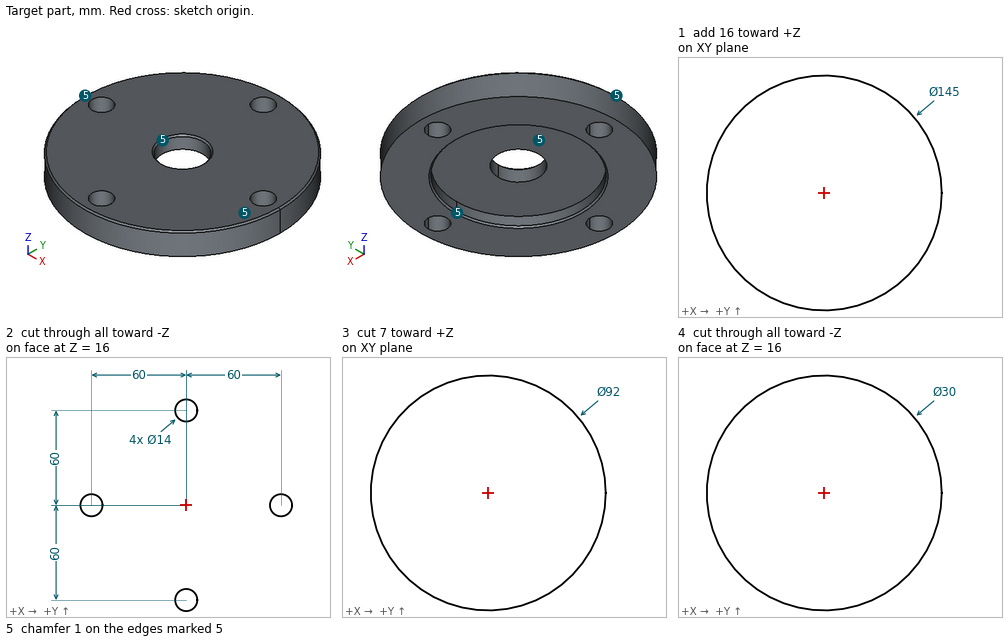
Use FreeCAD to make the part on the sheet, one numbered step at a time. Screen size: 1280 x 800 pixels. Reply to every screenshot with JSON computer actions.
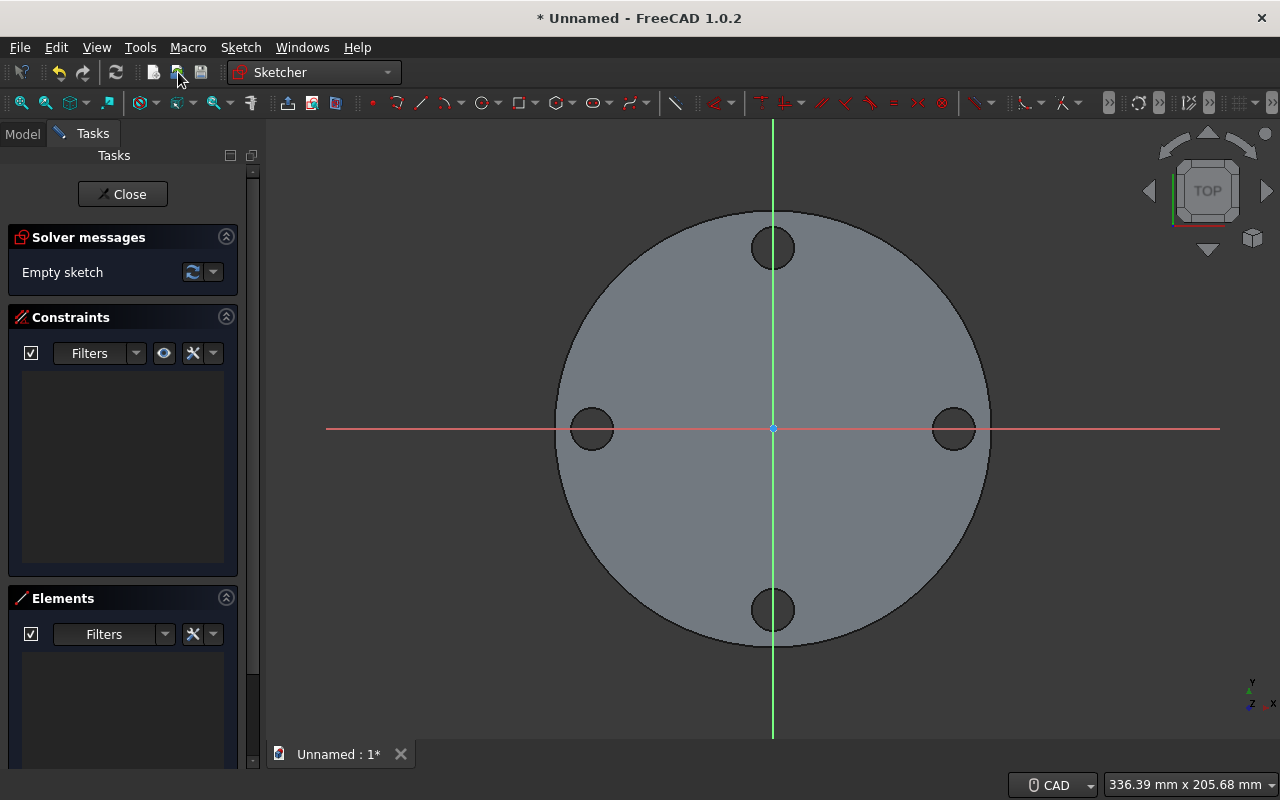
{"action": "scroll", "coordinate": [795, 429], "scroll_direction": "up", "scroll_amount": 7}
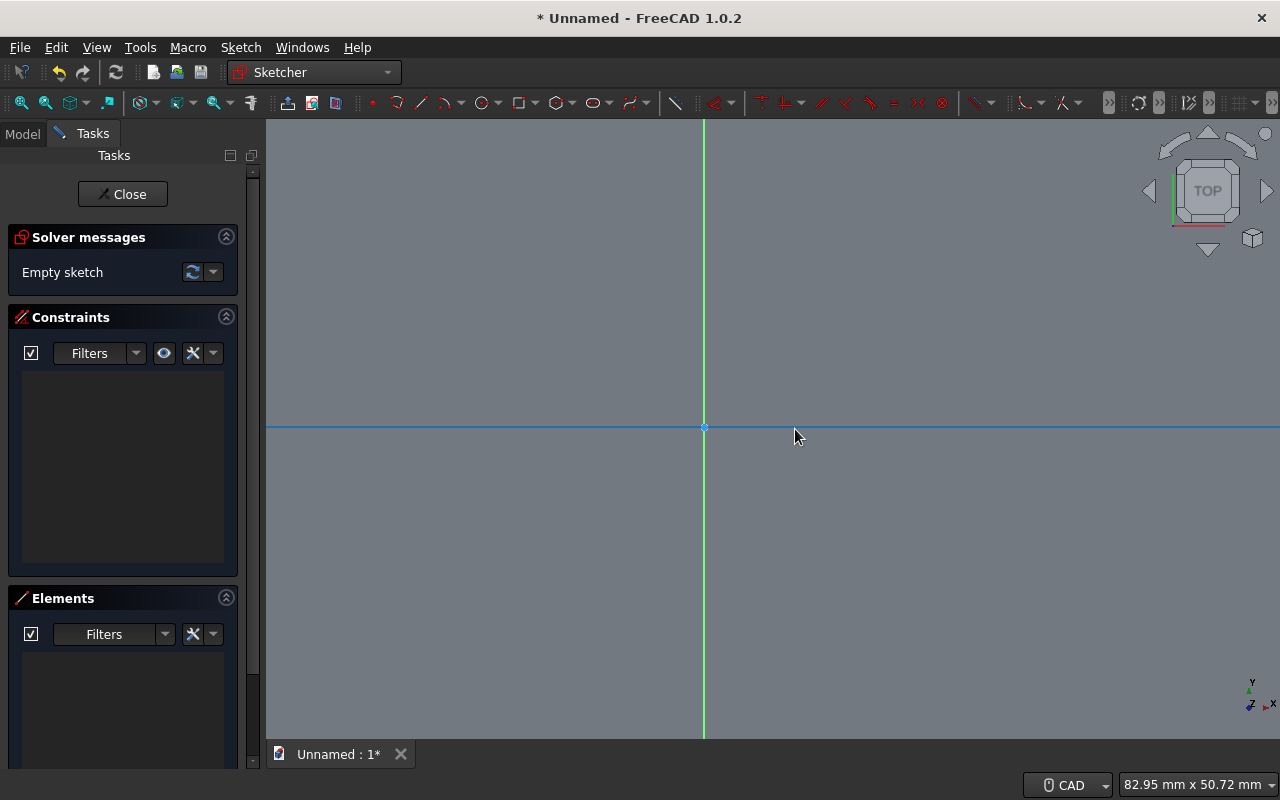
{"action": "key", "text": "g c"}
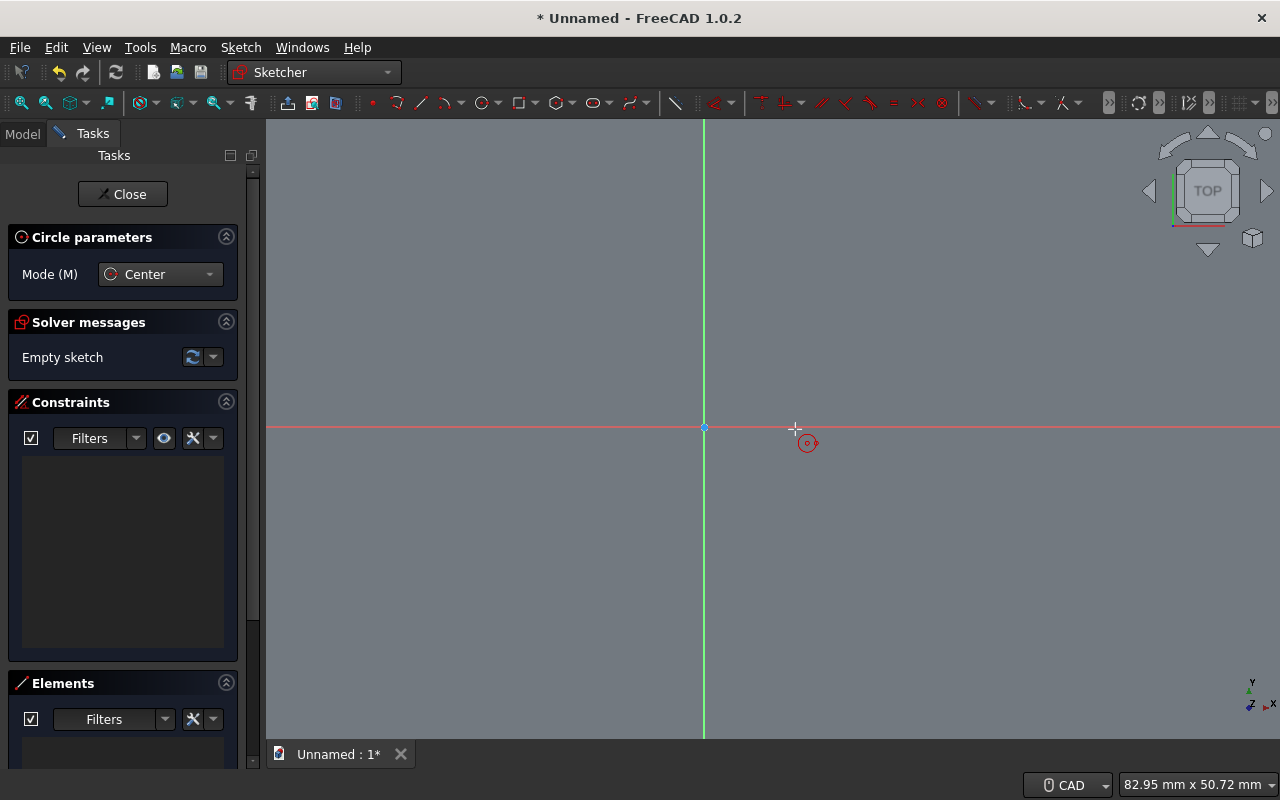
{"action": "left_click", "coordinate": [704, 427]}
{"action": "left_click", "coordinate": [834, 298]}
{"action": "key", "text": "Escape"}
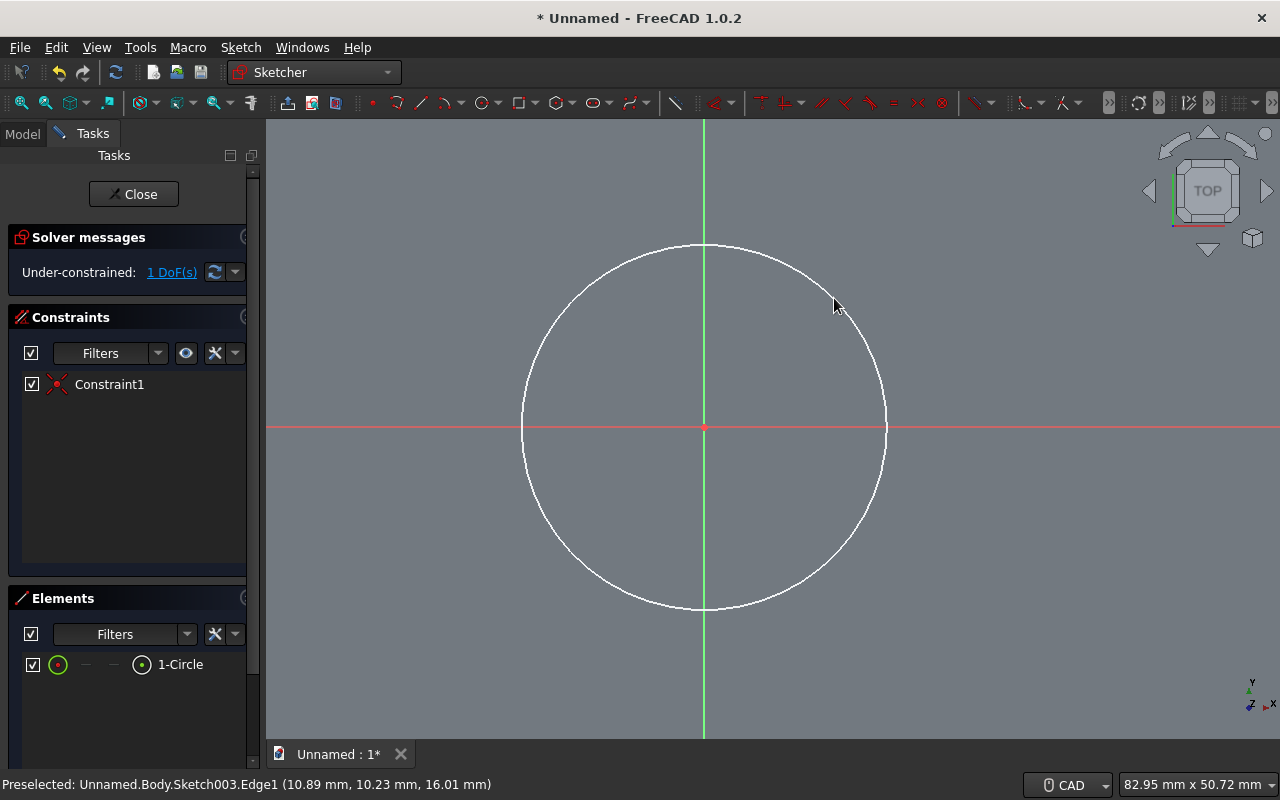
{"action": "key", "text": "d"}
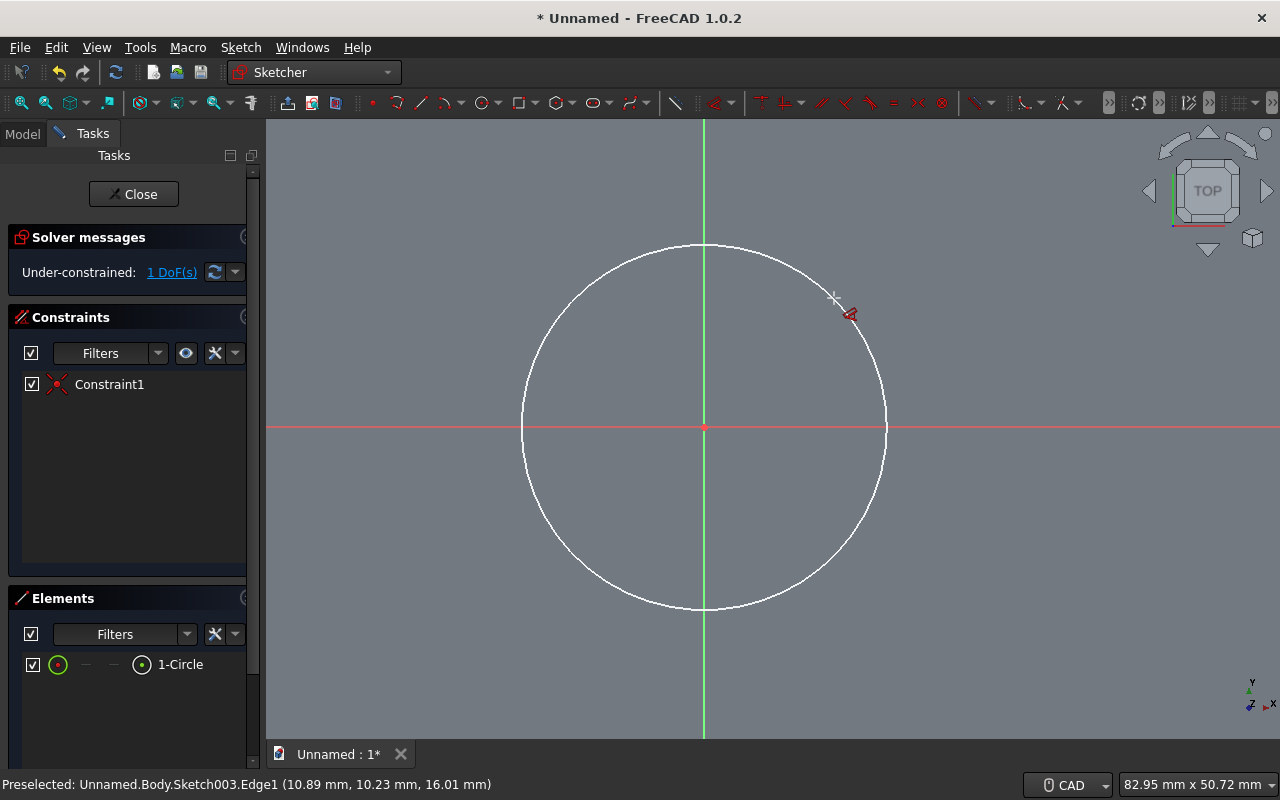
{"action": "left_click", "coordinate": [833, 298]}
{"action": "left_click", "coordinate": [856, 275]}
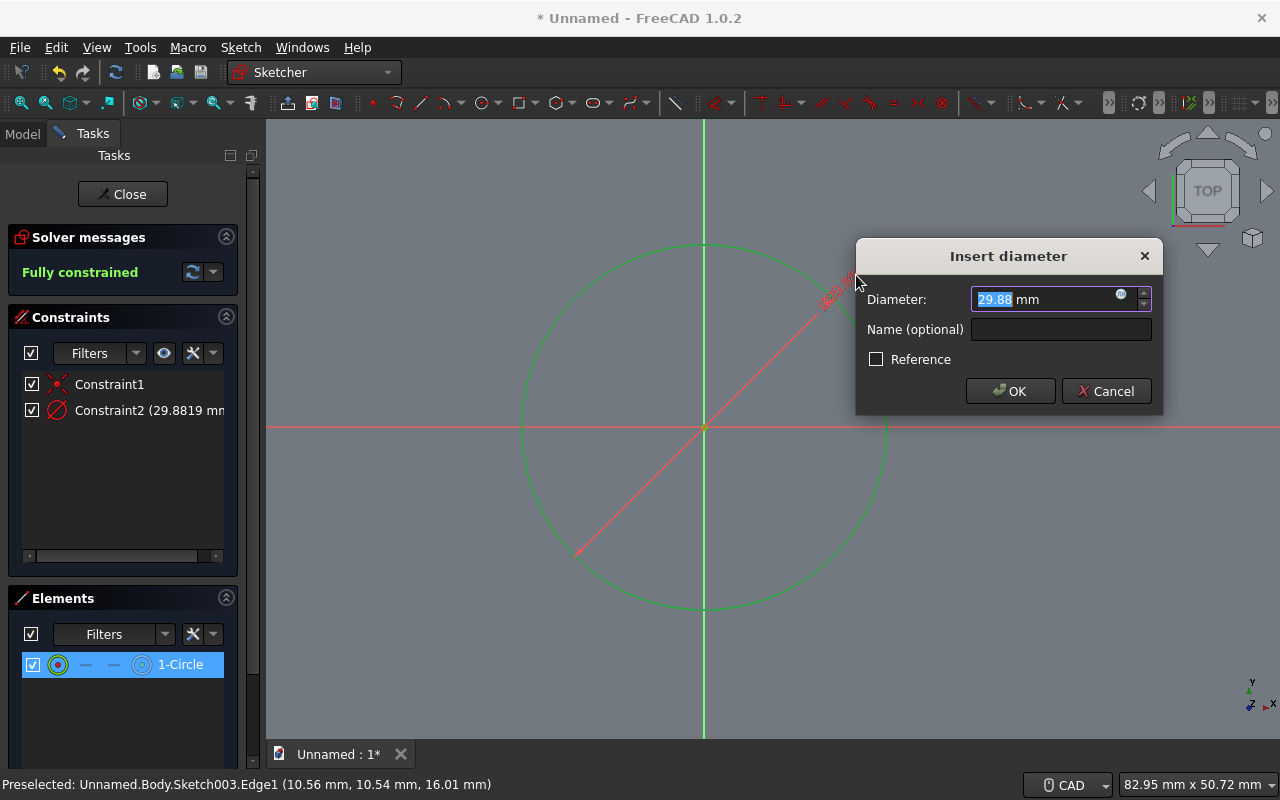
{"action": "type", "text": "30"}
{"action": "key", "text": "Return"}
{"action": "key", "text": "Escape"}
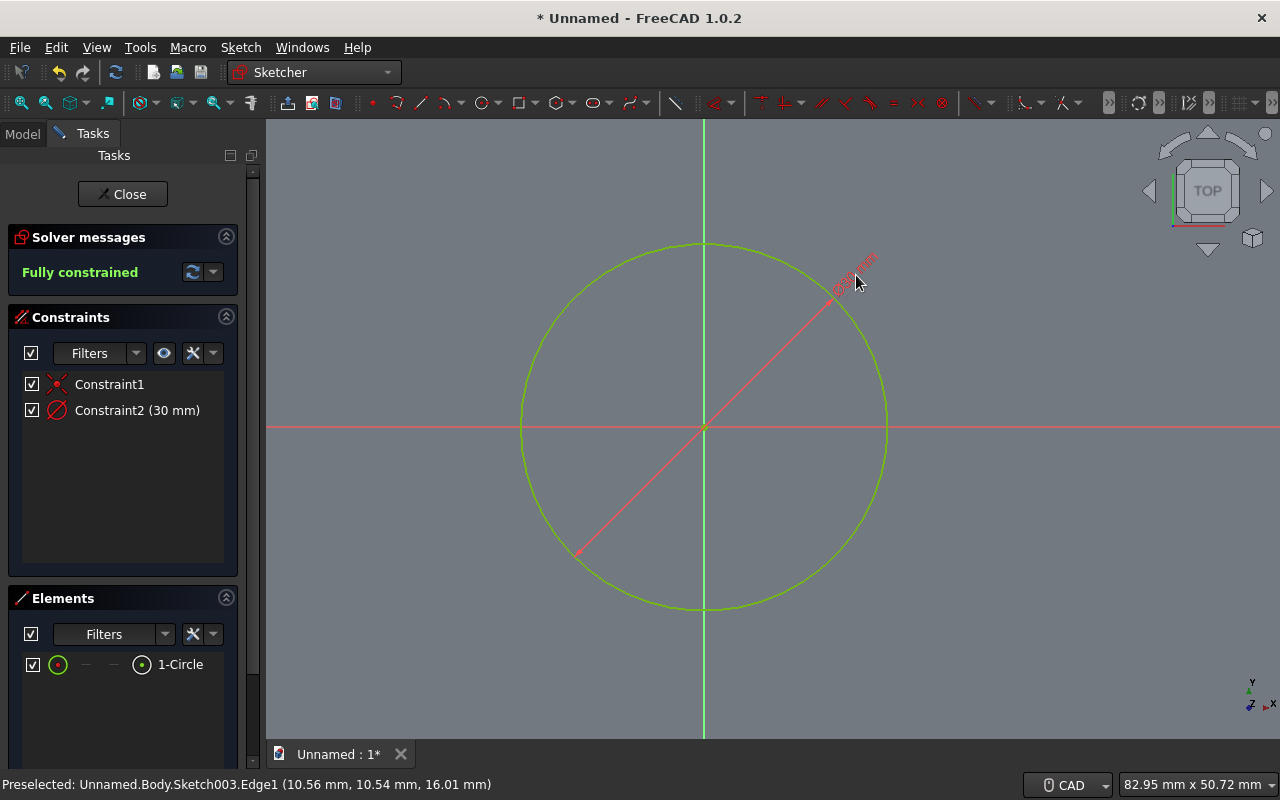
{"action": "left_click", "coordinate": [123, 194]}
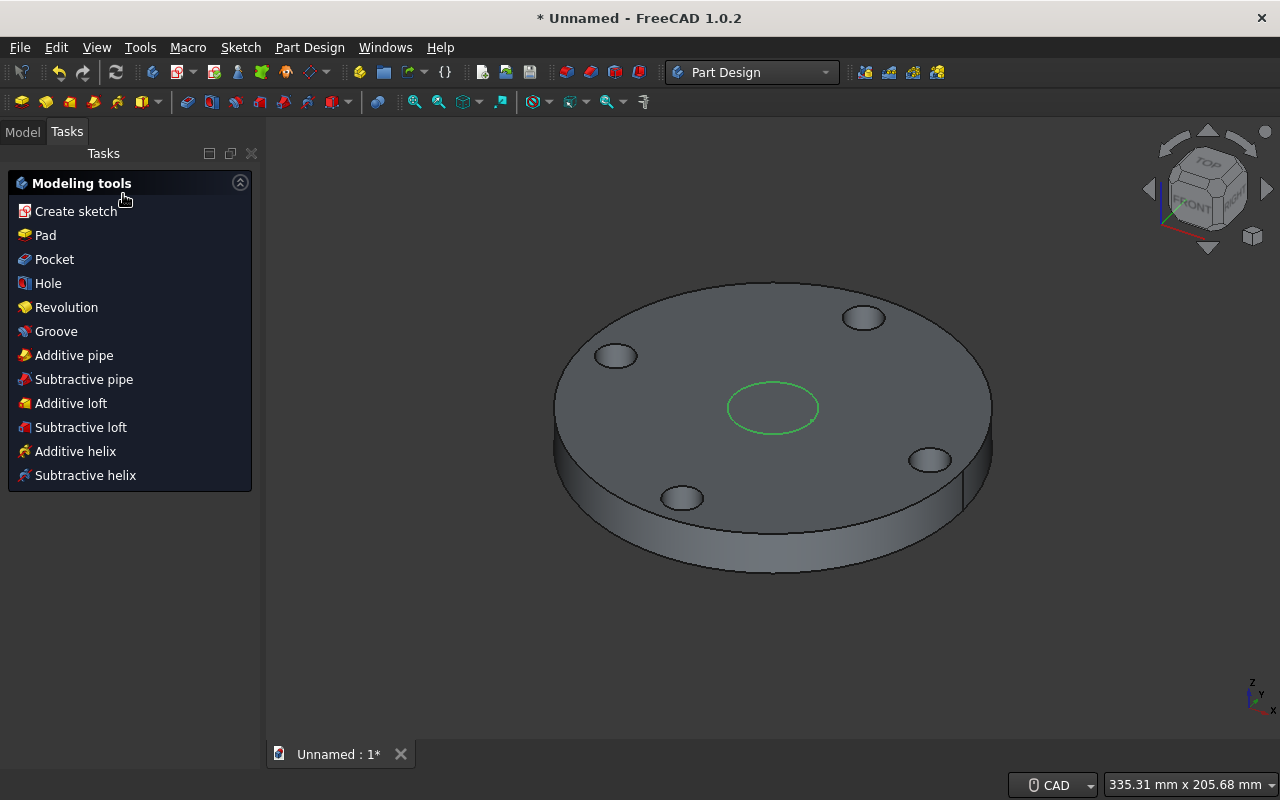
{"action": "left_click", "coordinate": [188, 102]}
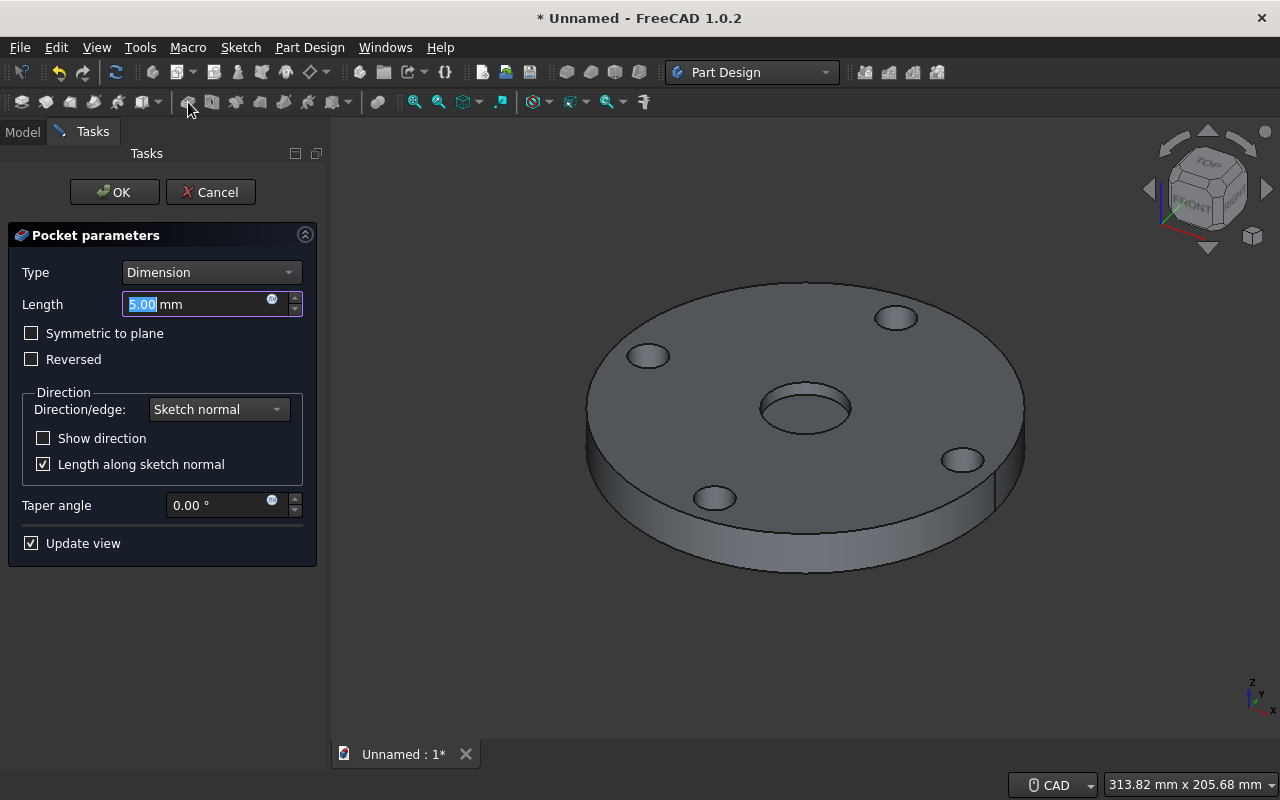
{"action": "left_click", "coordinate": [212, 272]}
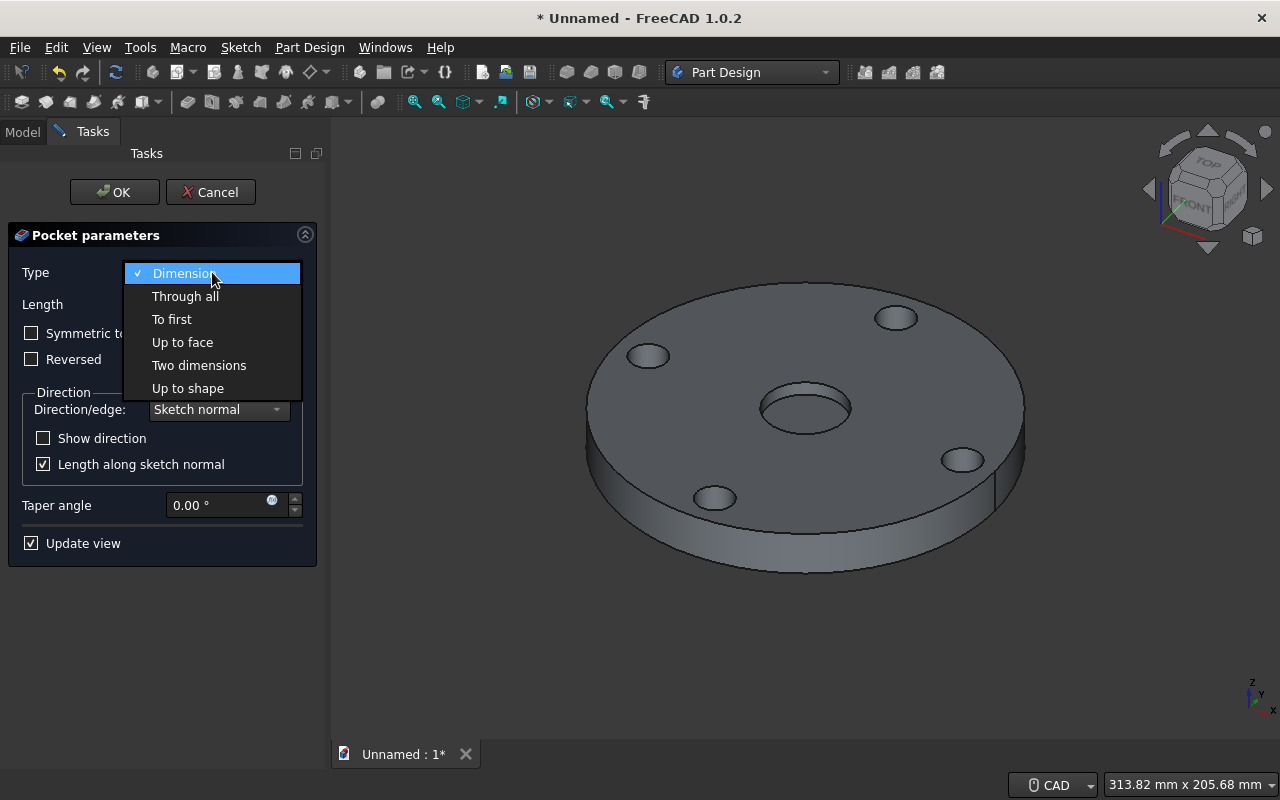
{"action": "left_click", "coordinate": [212, 296]}